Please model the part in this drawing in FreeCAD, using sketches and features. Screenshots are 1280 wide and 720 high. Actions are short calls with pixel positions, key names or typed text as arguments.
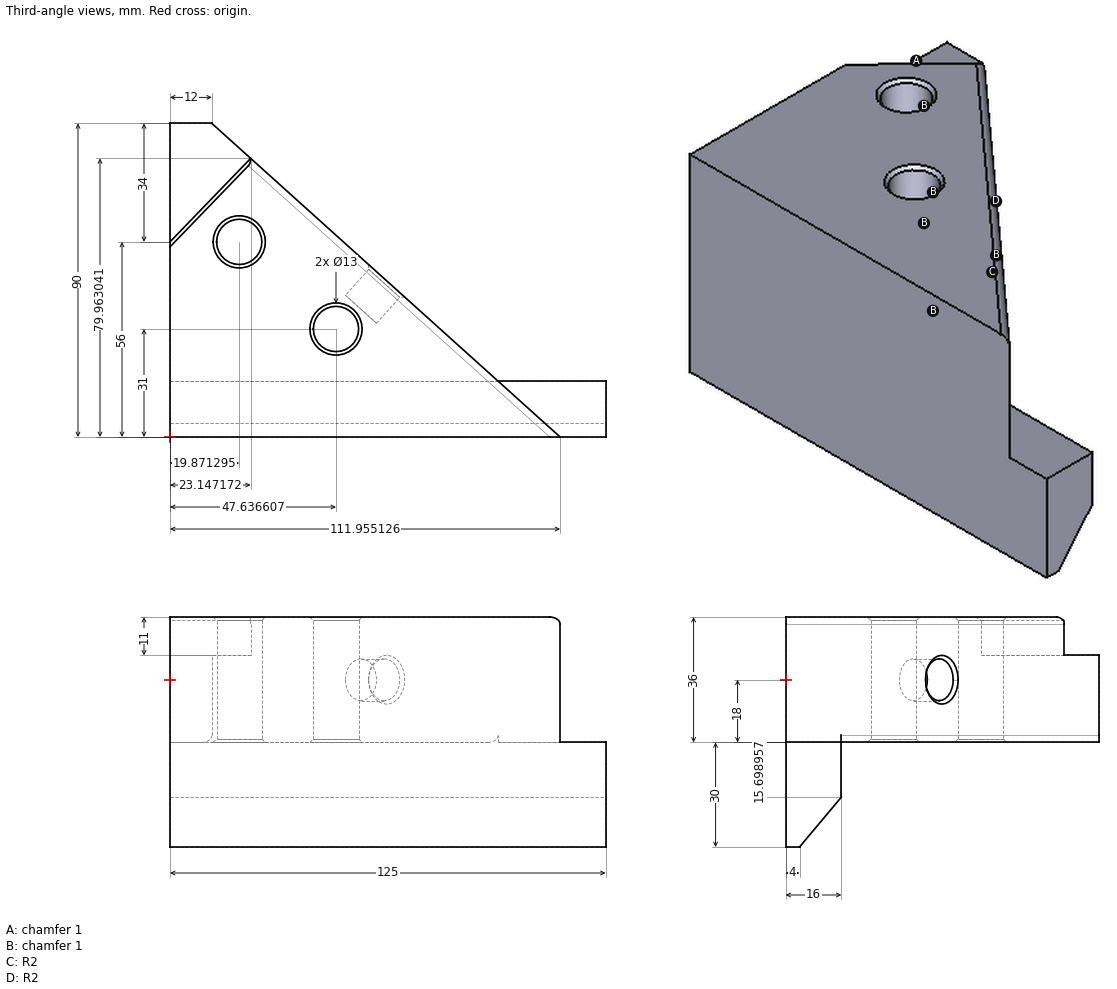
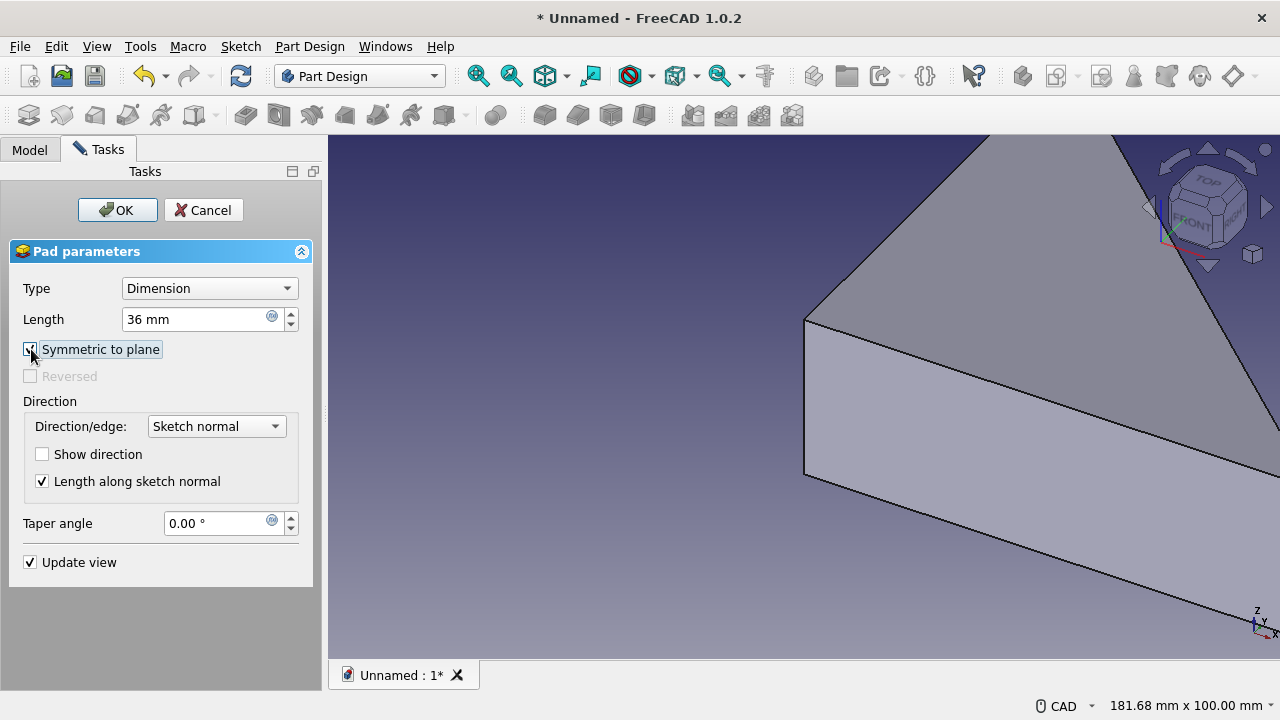
click(118, 210)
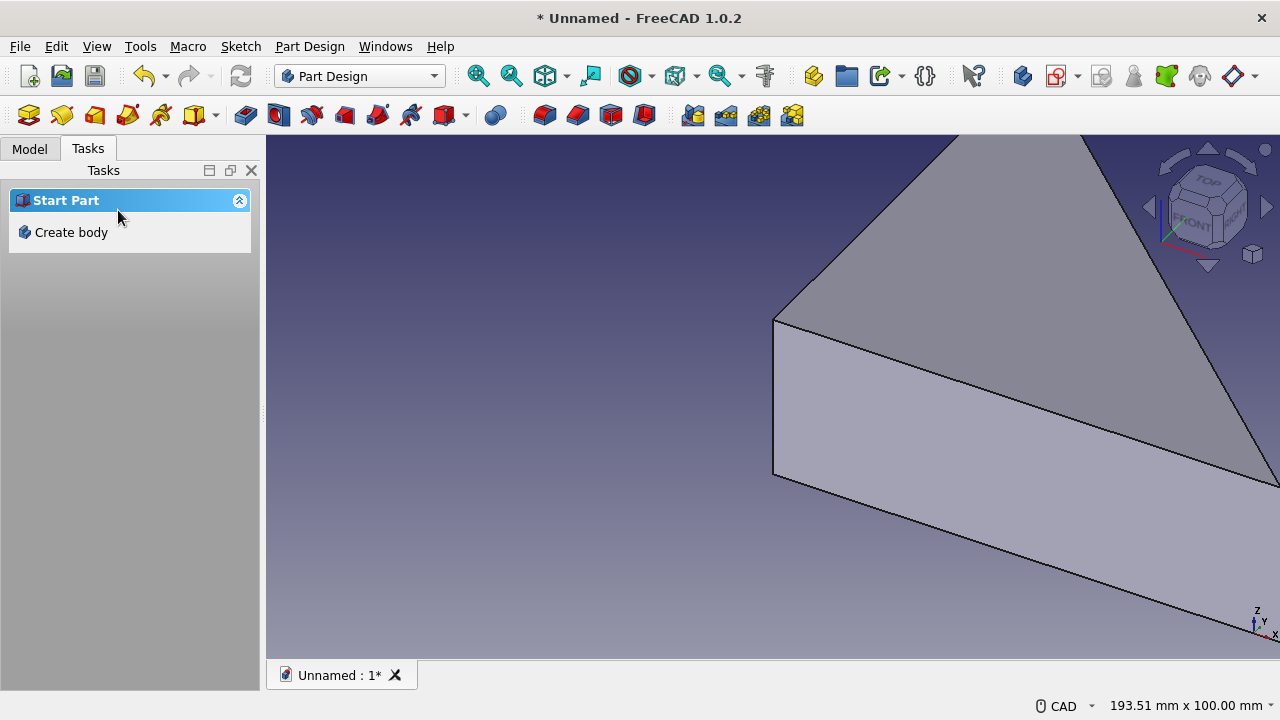
click(479, 76)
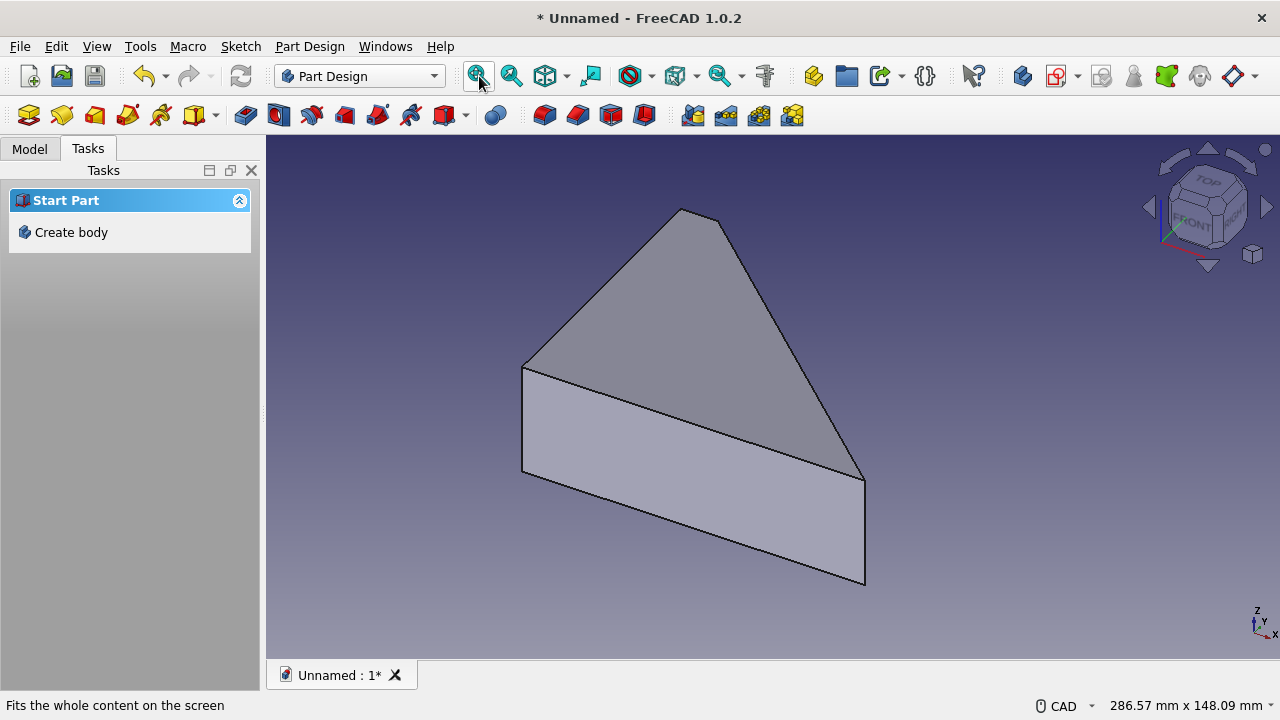
click(701, 350)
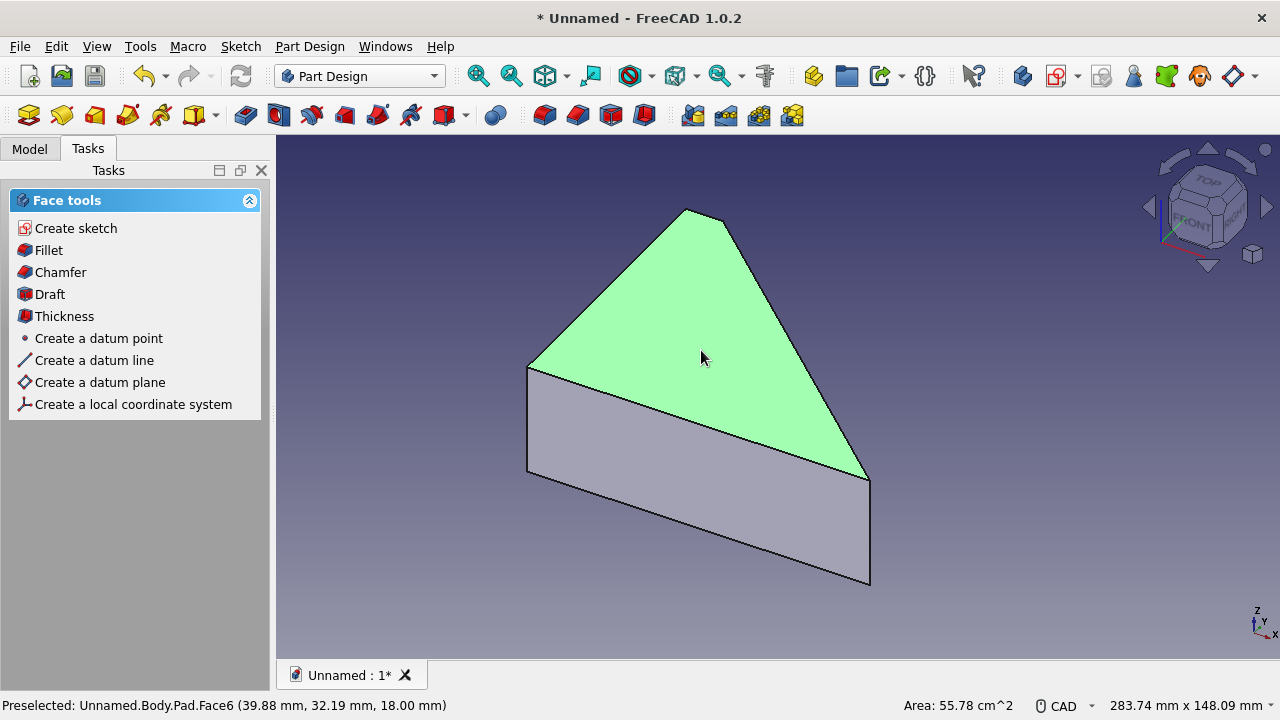
click(1056, 76)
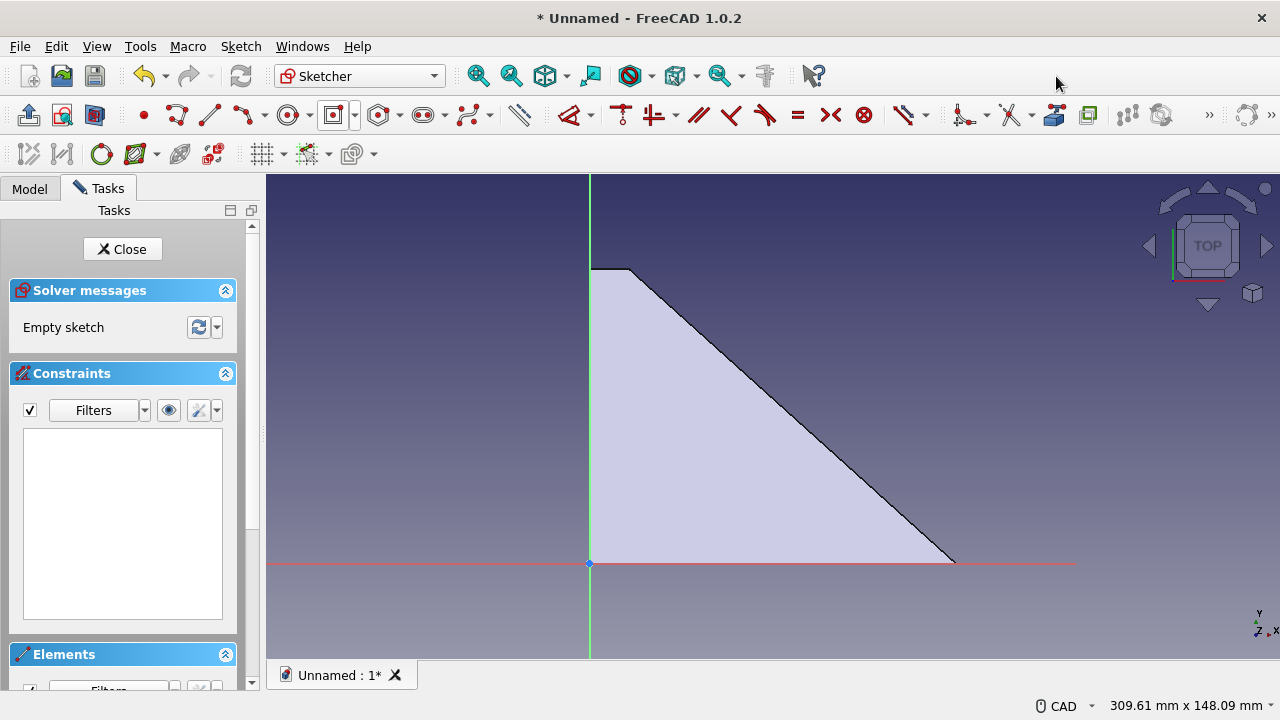
scroll(583, 271, up, 5)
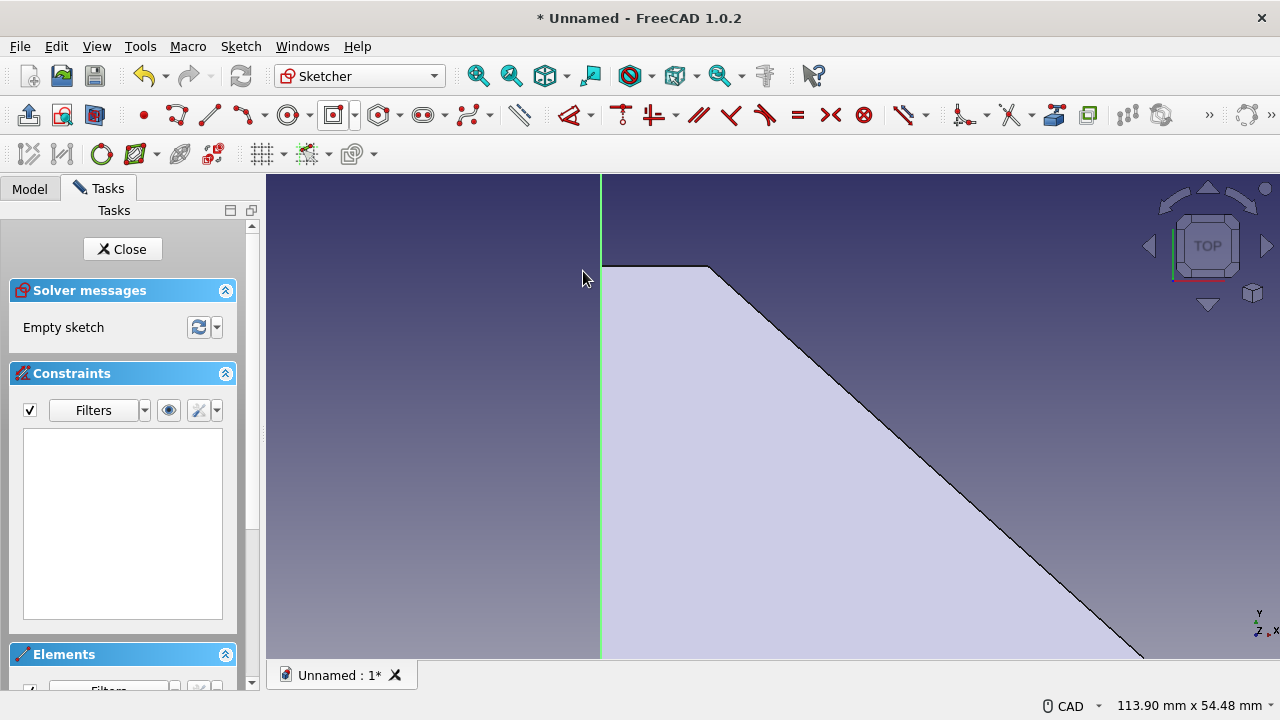
click(177, 116)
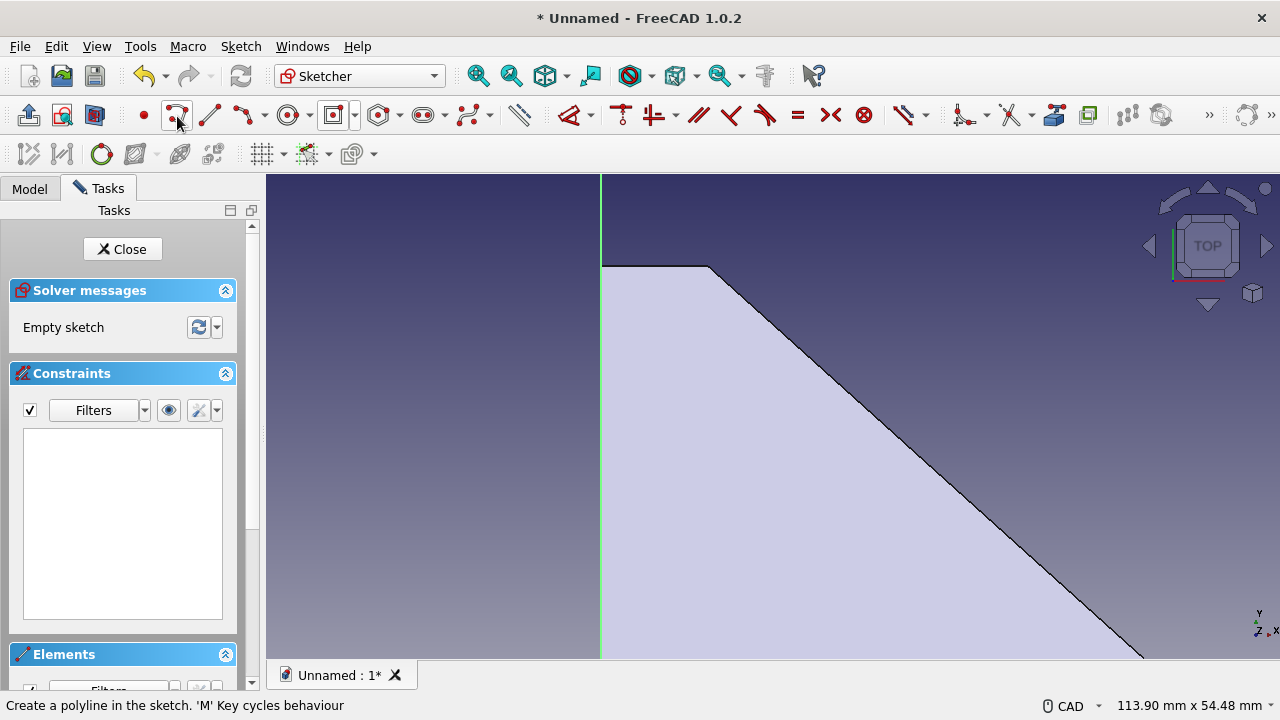
click(601, 568)
click(807, 355)
click(707, 266)
click(610, 266)
click(601, 569)
key(Escape)
key(Escape)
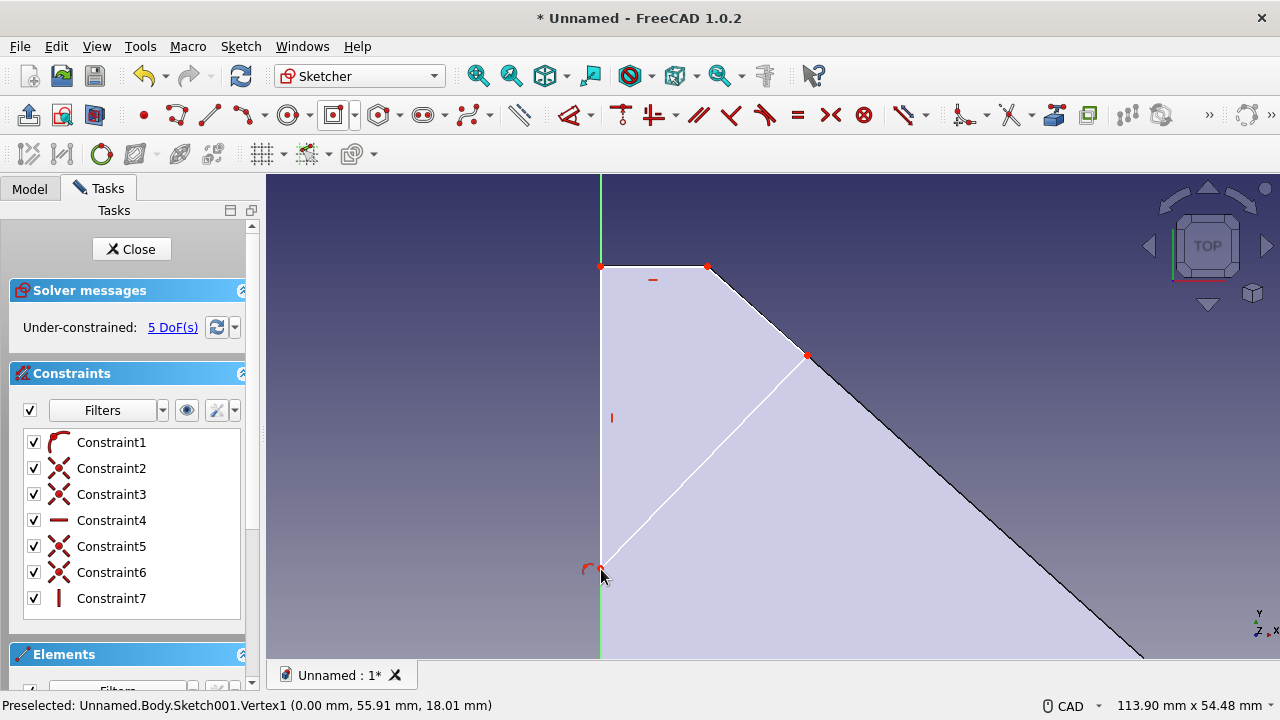
click(568, 116)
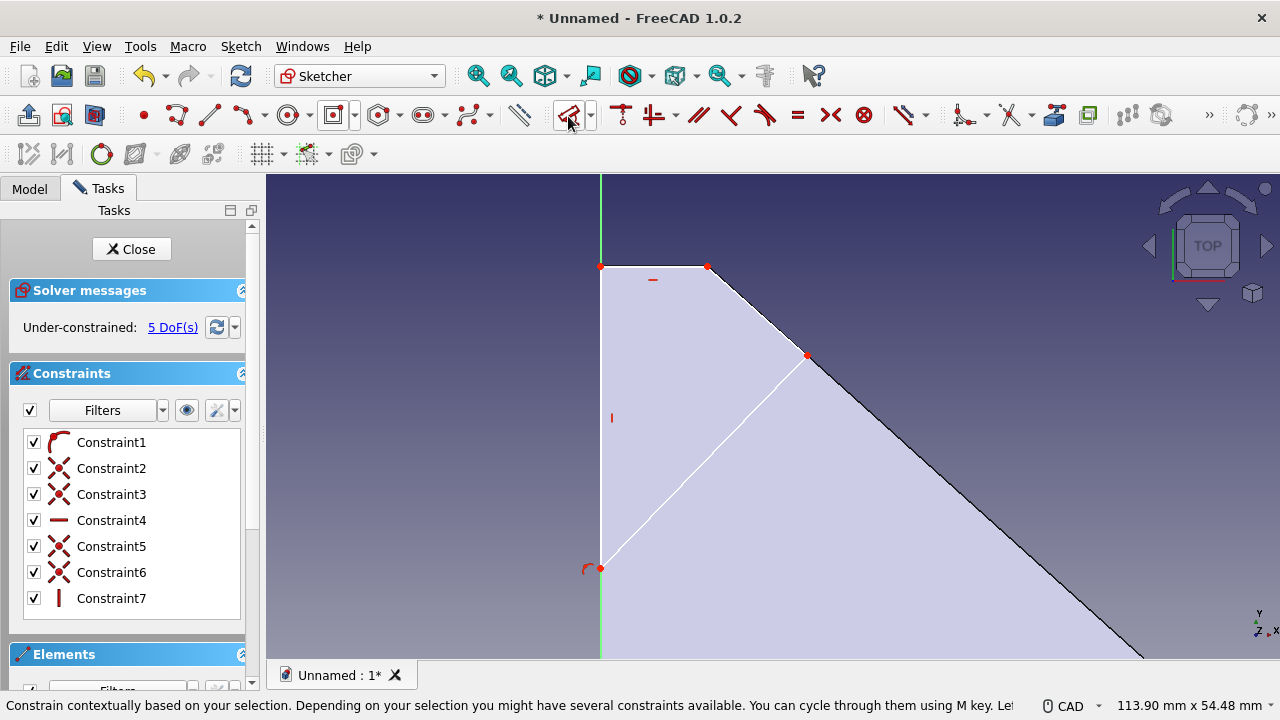
click(675, 267)
click(654, 233)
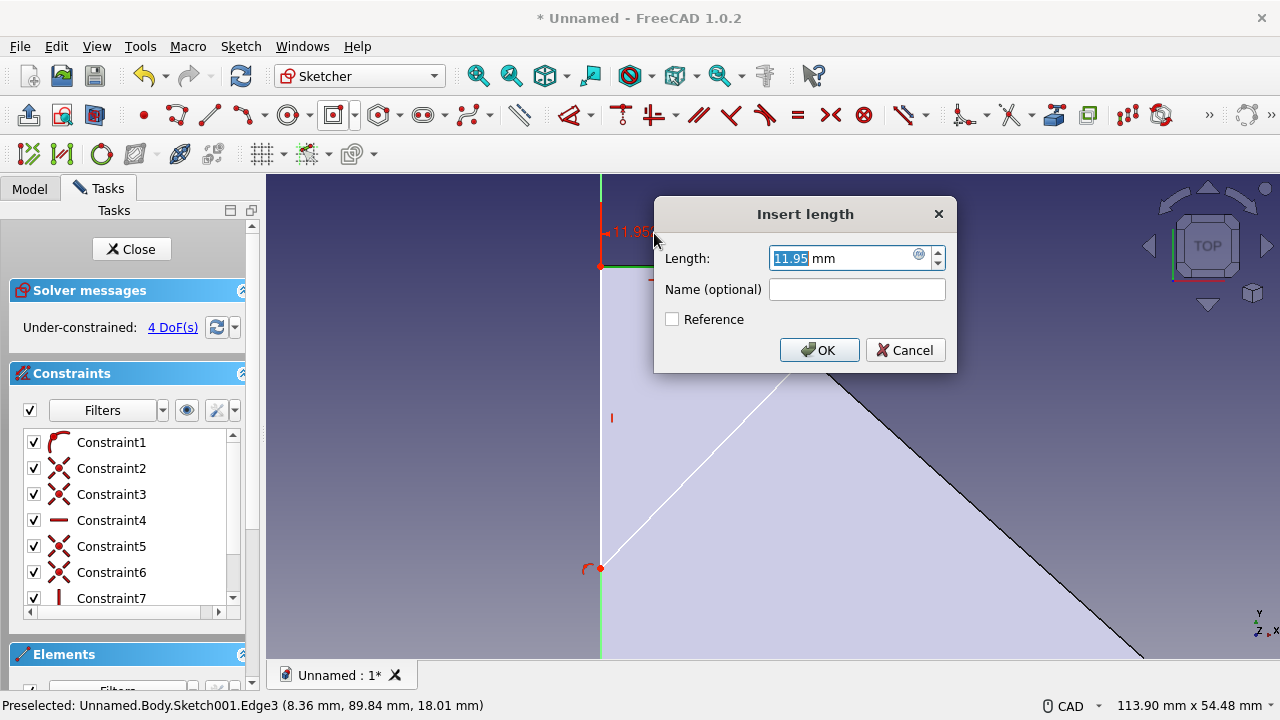
text(12)
key(Return)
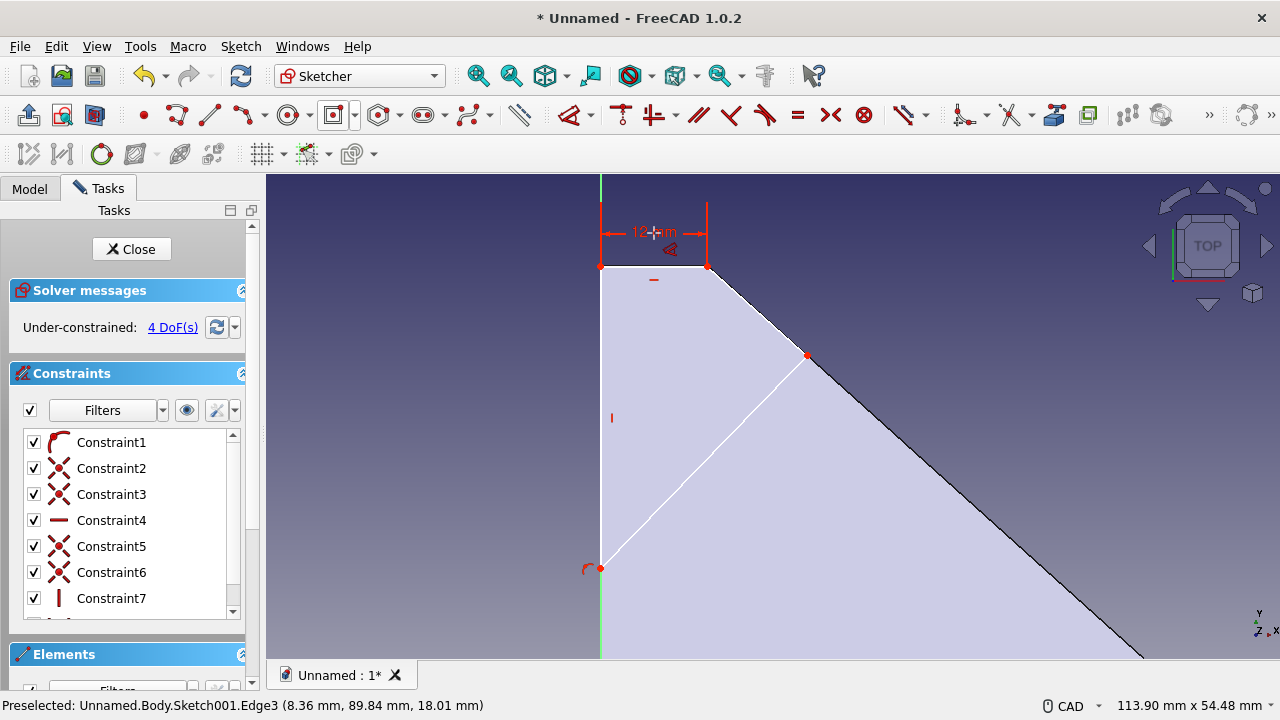
click(601, 358)
click(567, 418)